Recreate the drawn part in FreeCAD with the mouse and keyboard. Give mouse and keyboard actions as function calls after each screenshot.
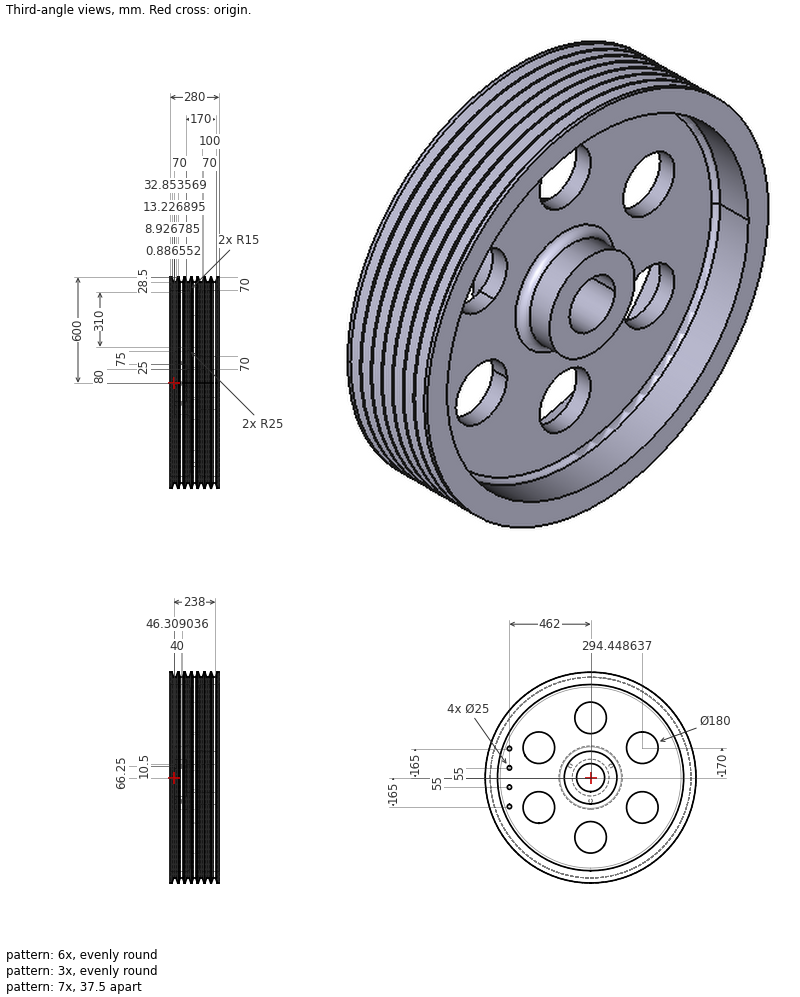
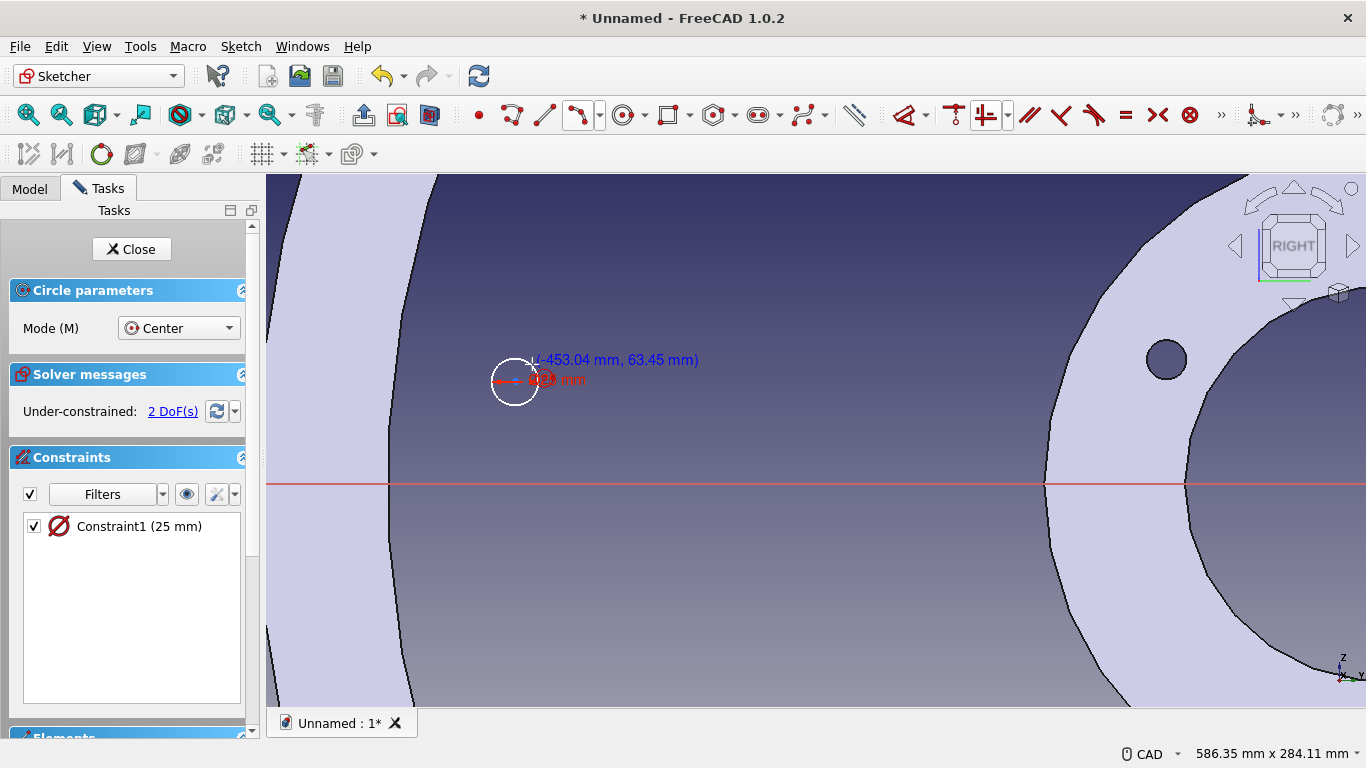
scroll(517, 388, down, 3)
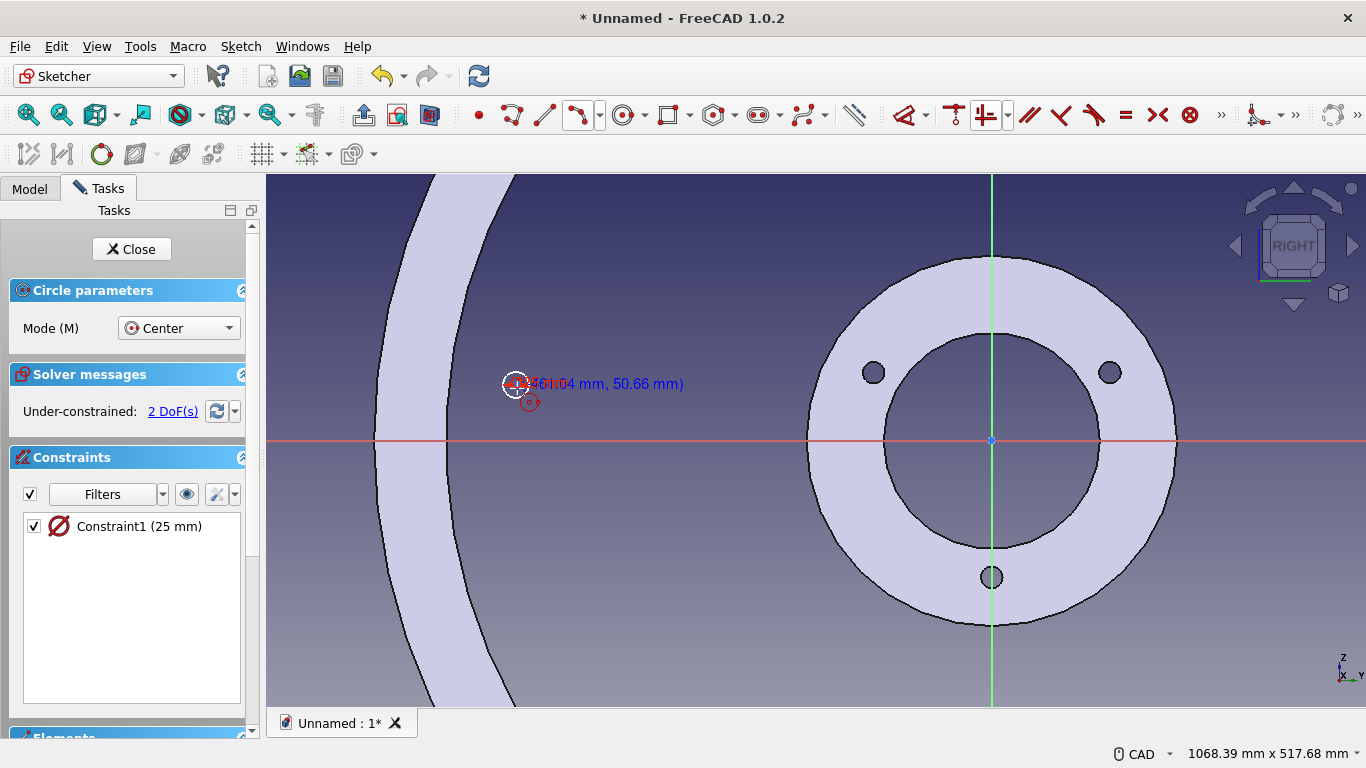
scroll(516, 271, up, 3)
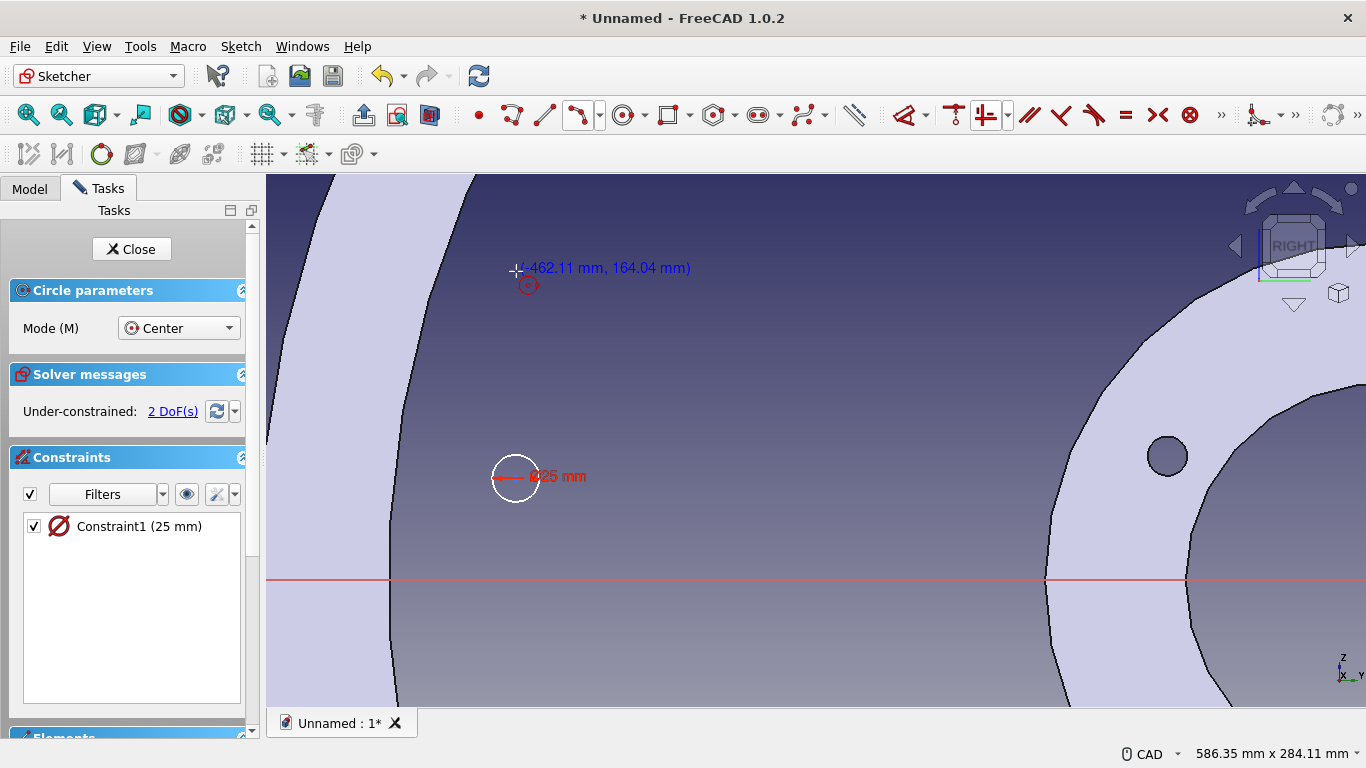
click(516, 271)
move(533, 254)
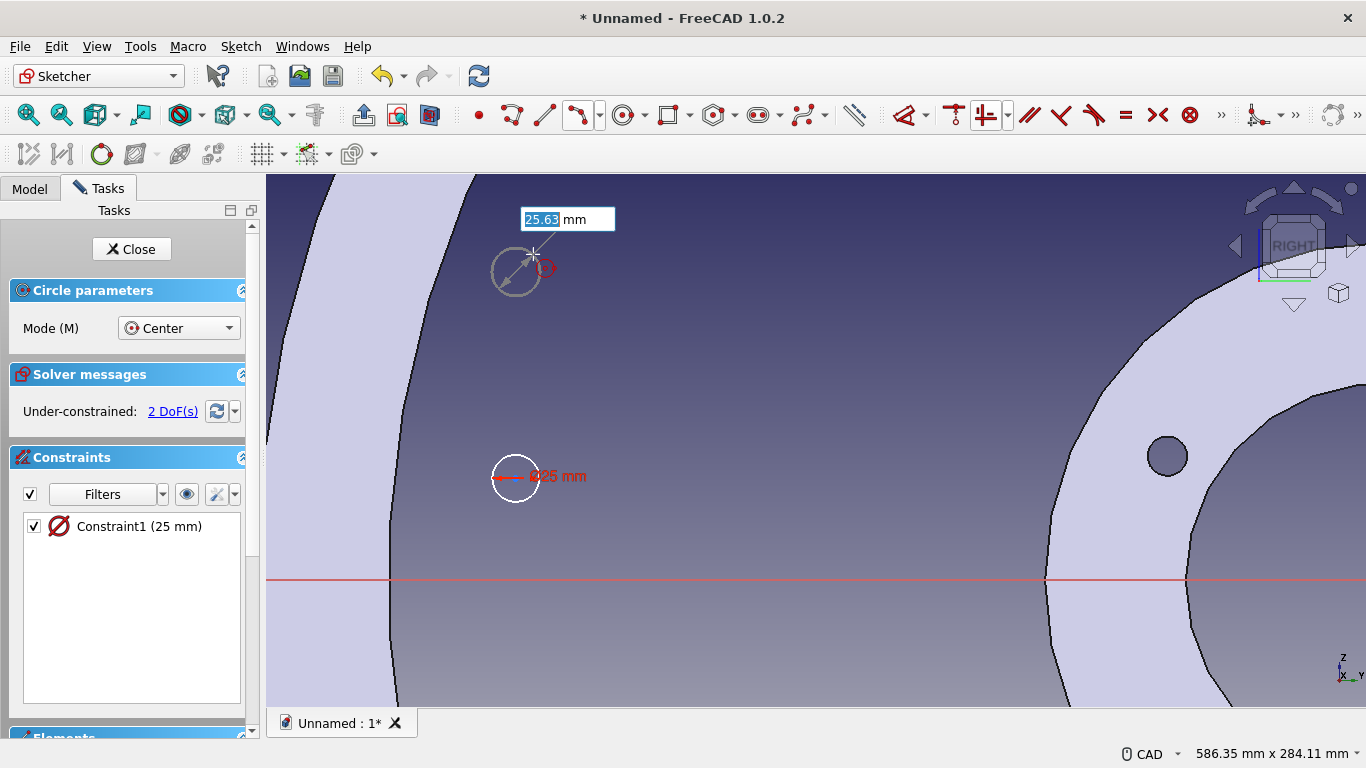
text(25)
key(Return)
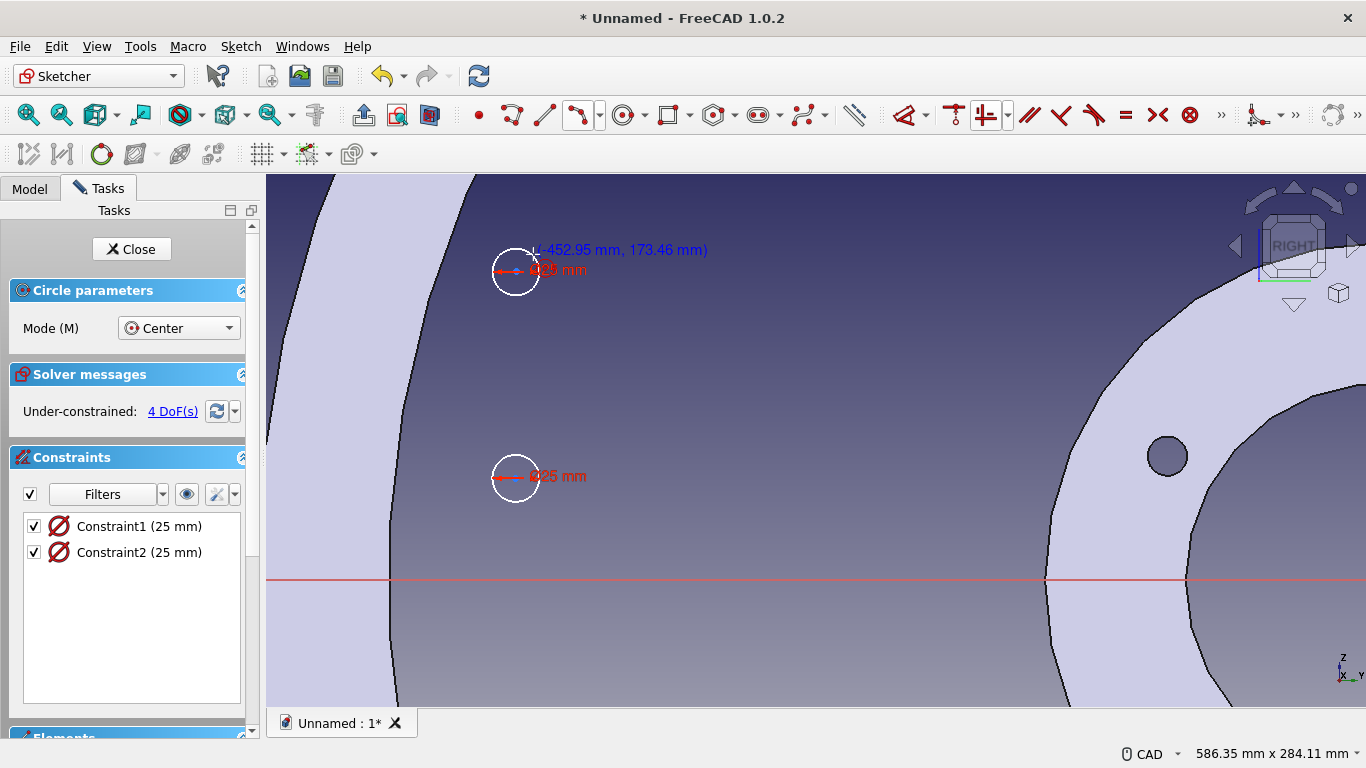
scroll(516, 270, down, 3)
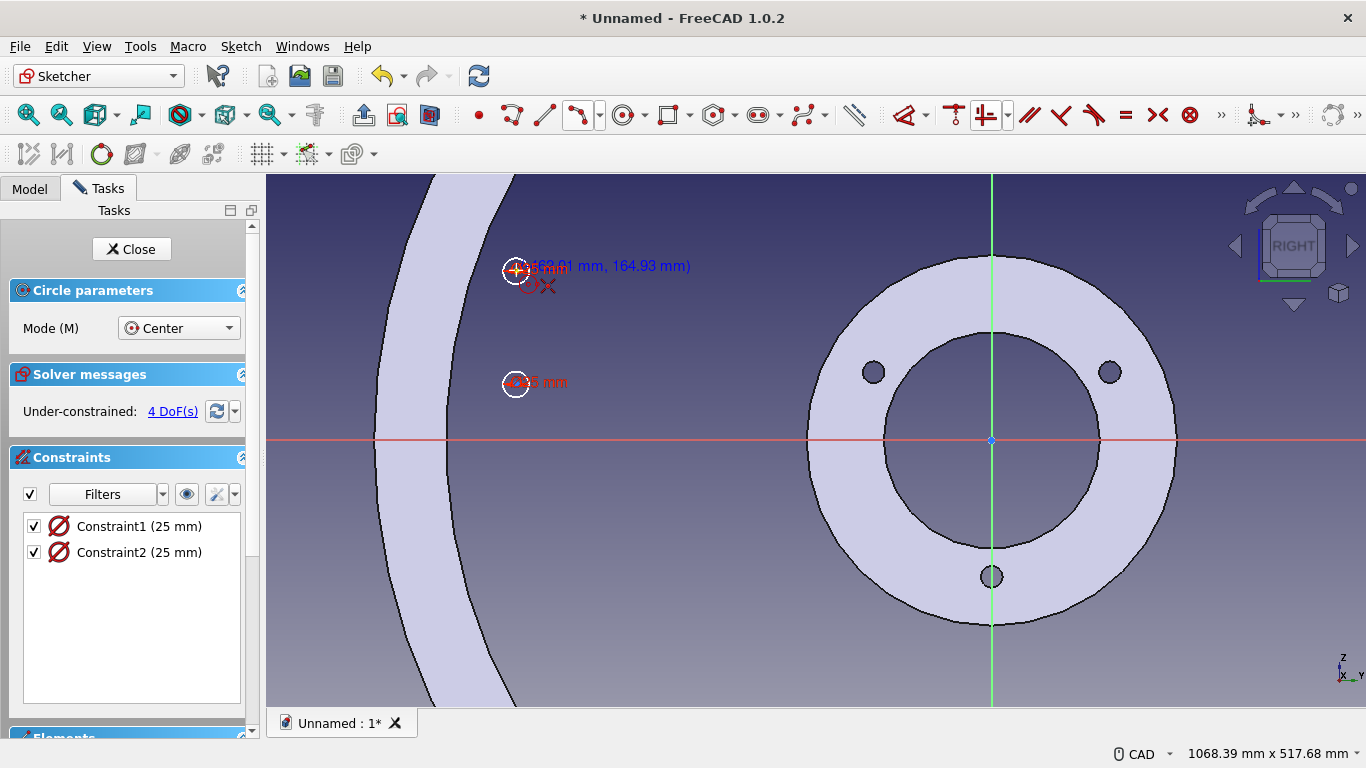
scroll(516, 497, up, 3)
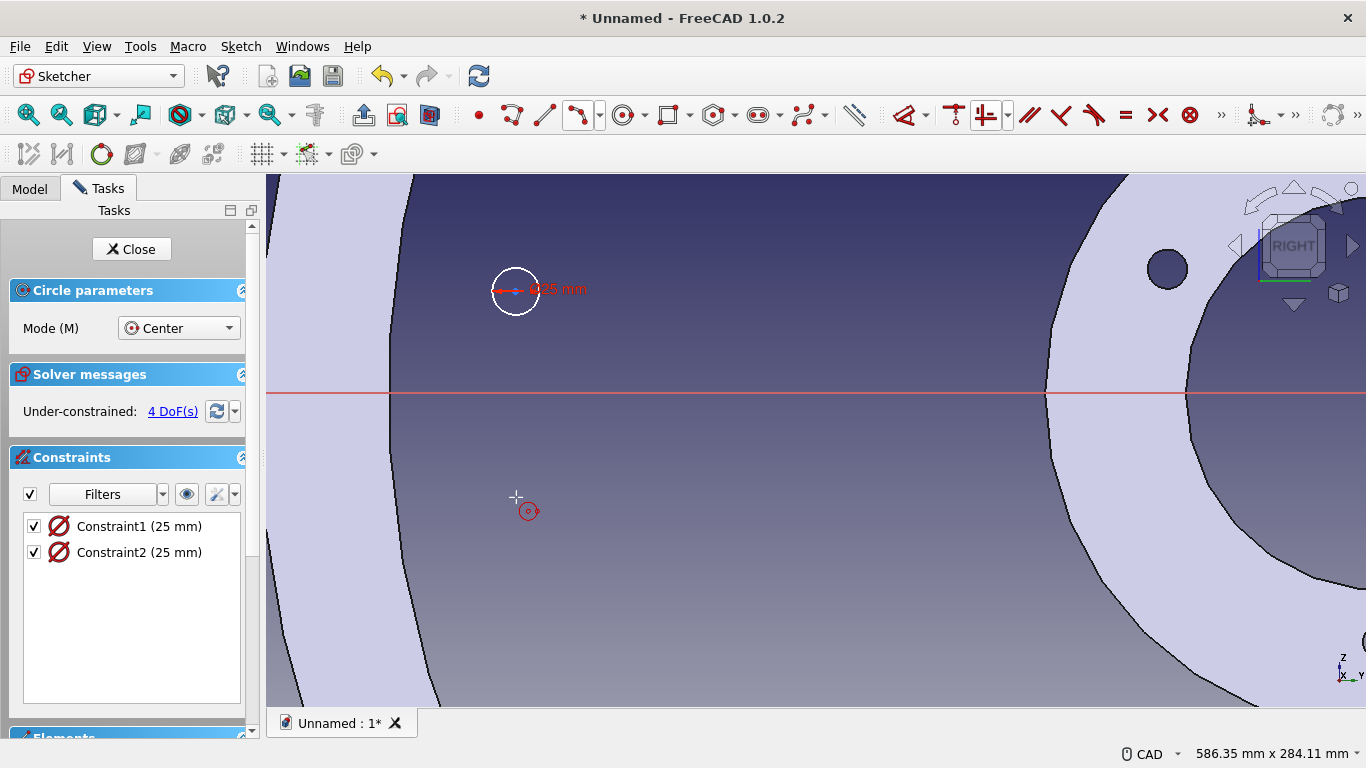
click(516, 497)
move(533, 480)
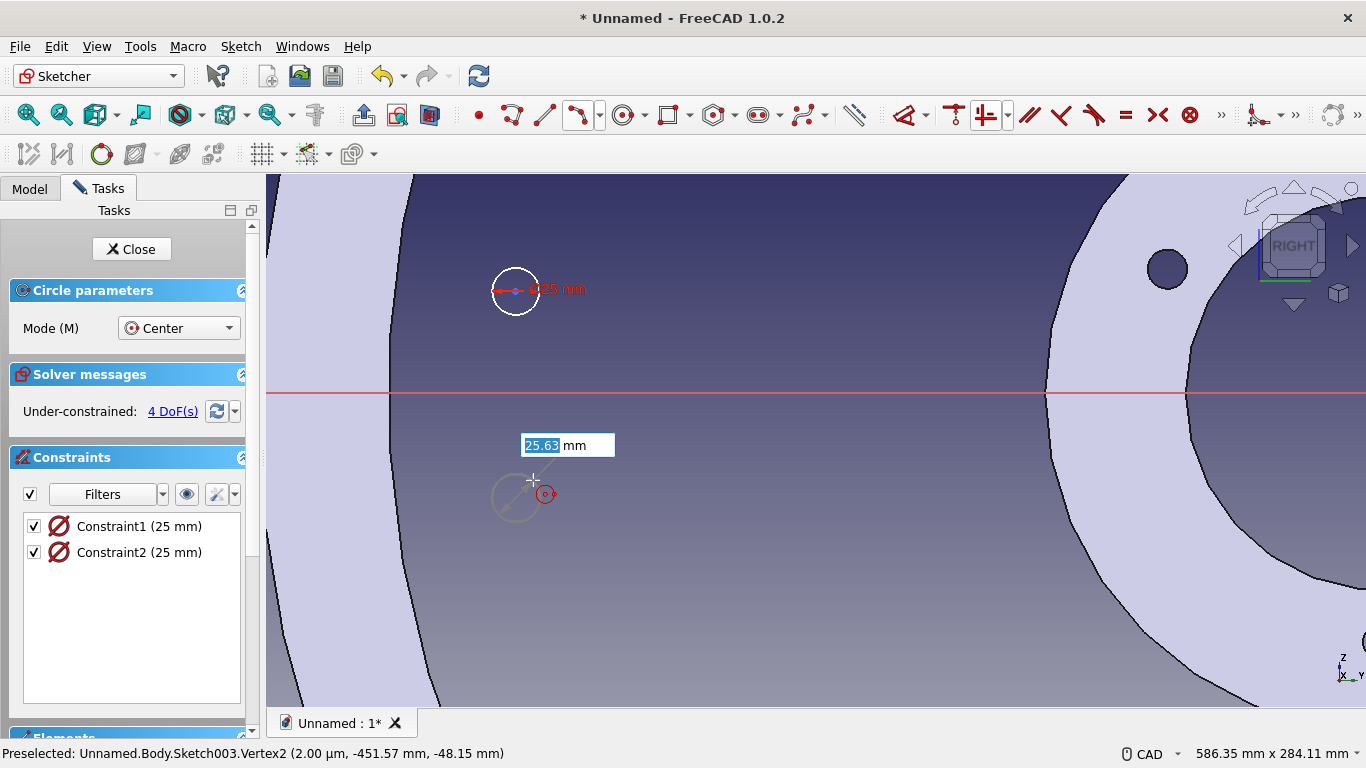
text(25)
key(Return)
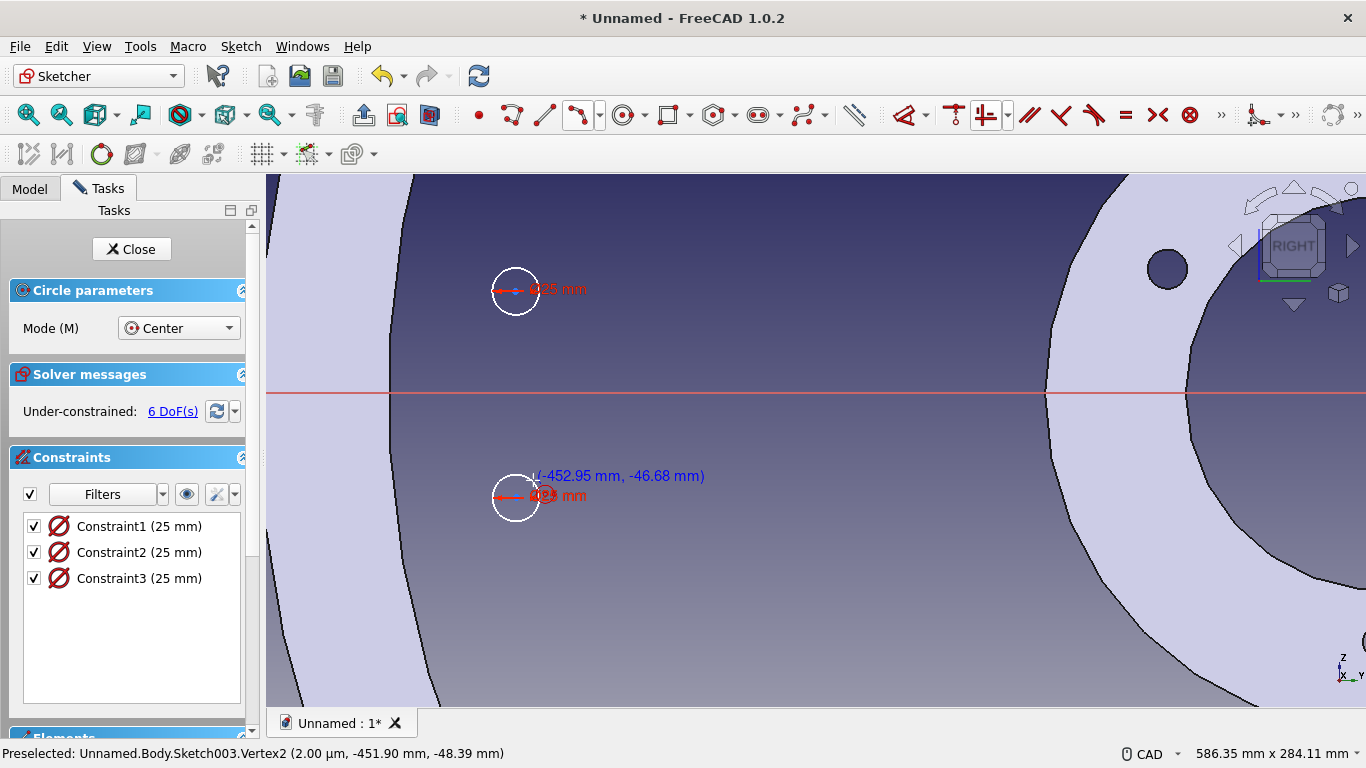
scroll(516, 498, down, 3)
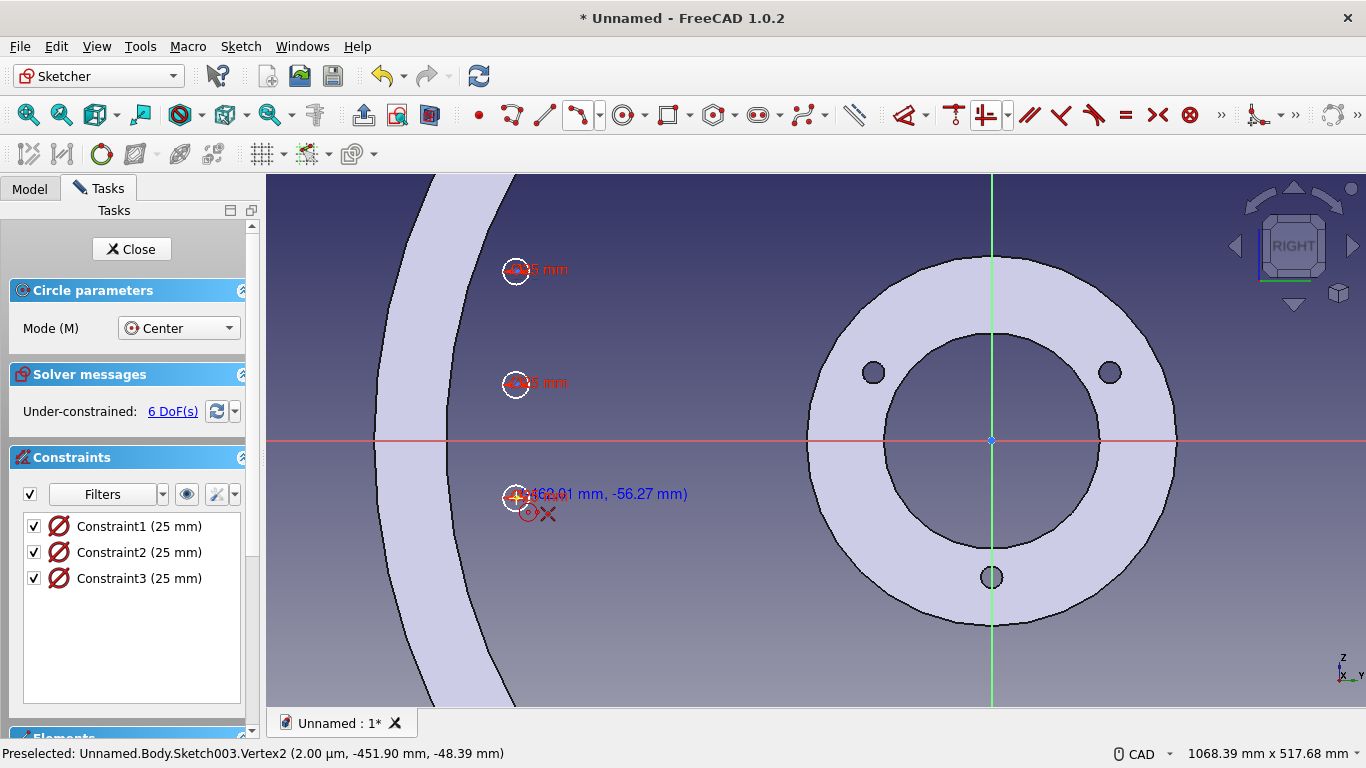
scroll(516, 611, up, 3)